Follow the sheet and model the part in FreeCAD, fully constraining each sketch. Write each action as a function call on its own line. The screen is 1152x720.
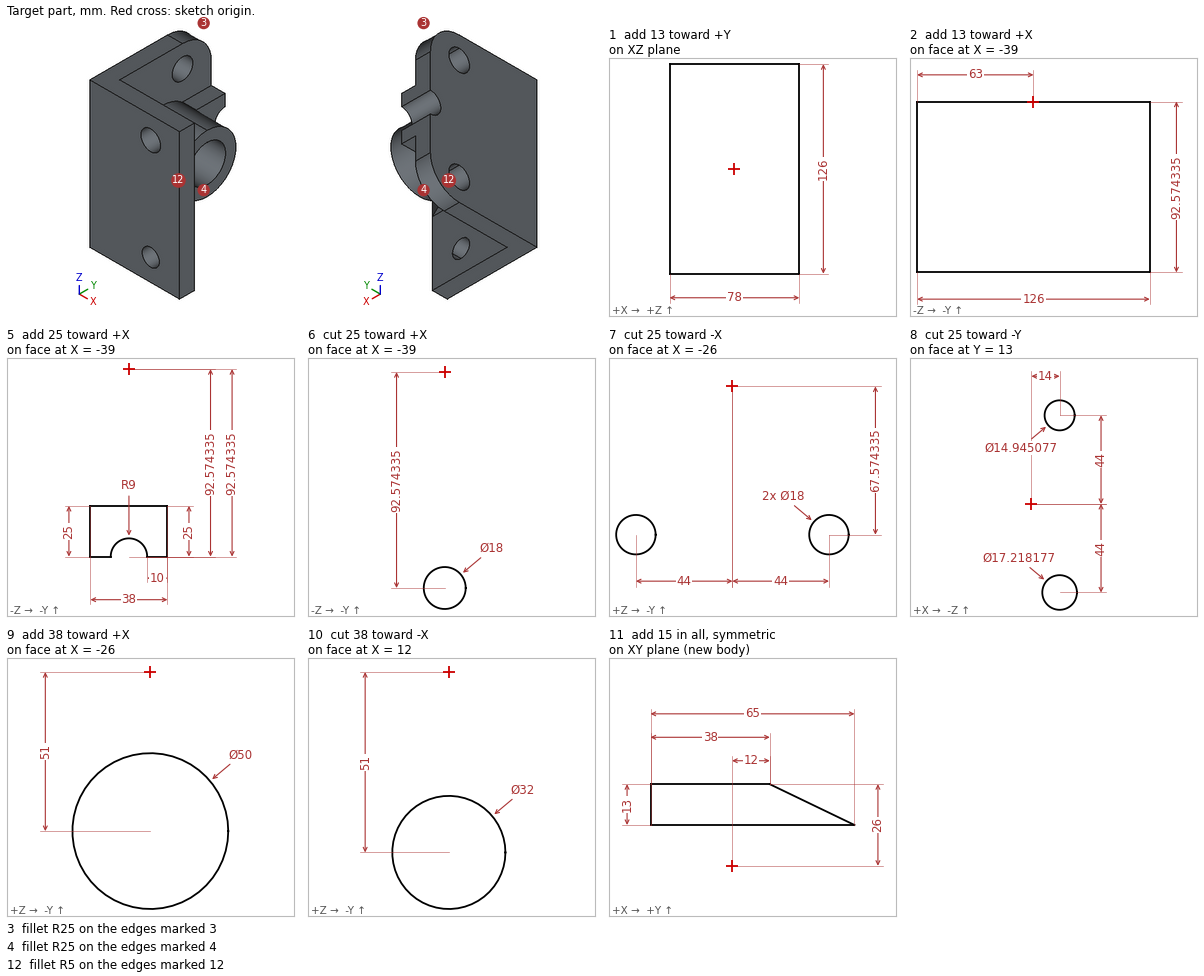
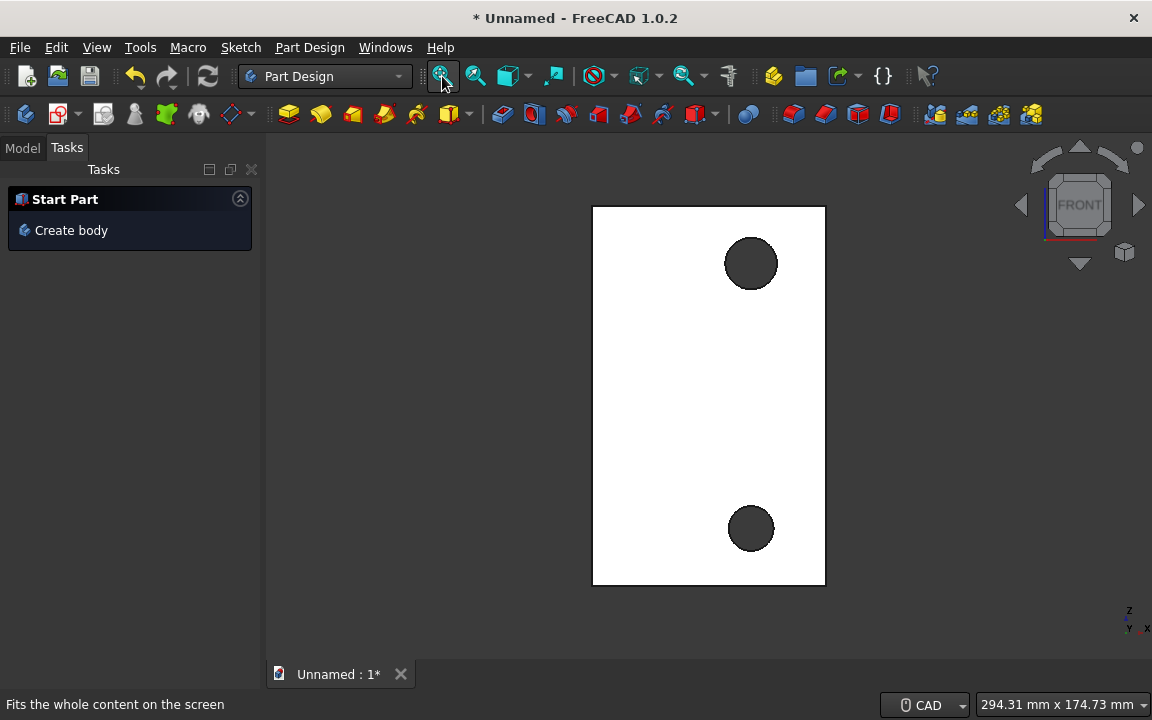
key(3)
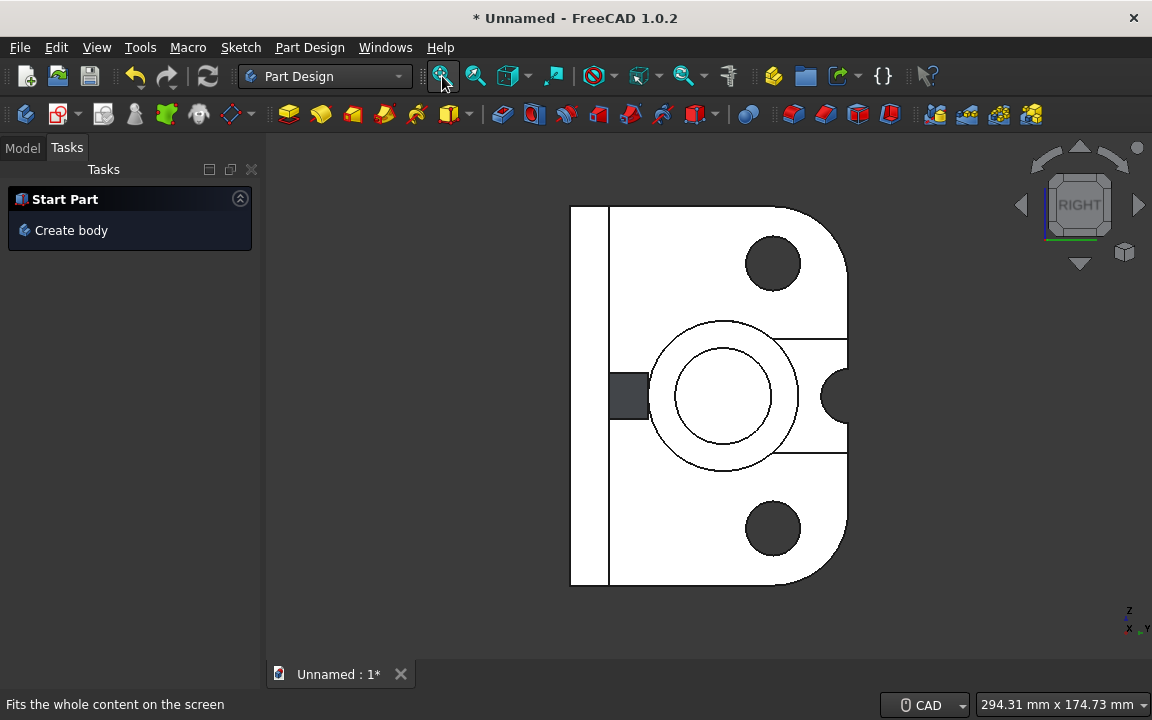
key(v)
key(f)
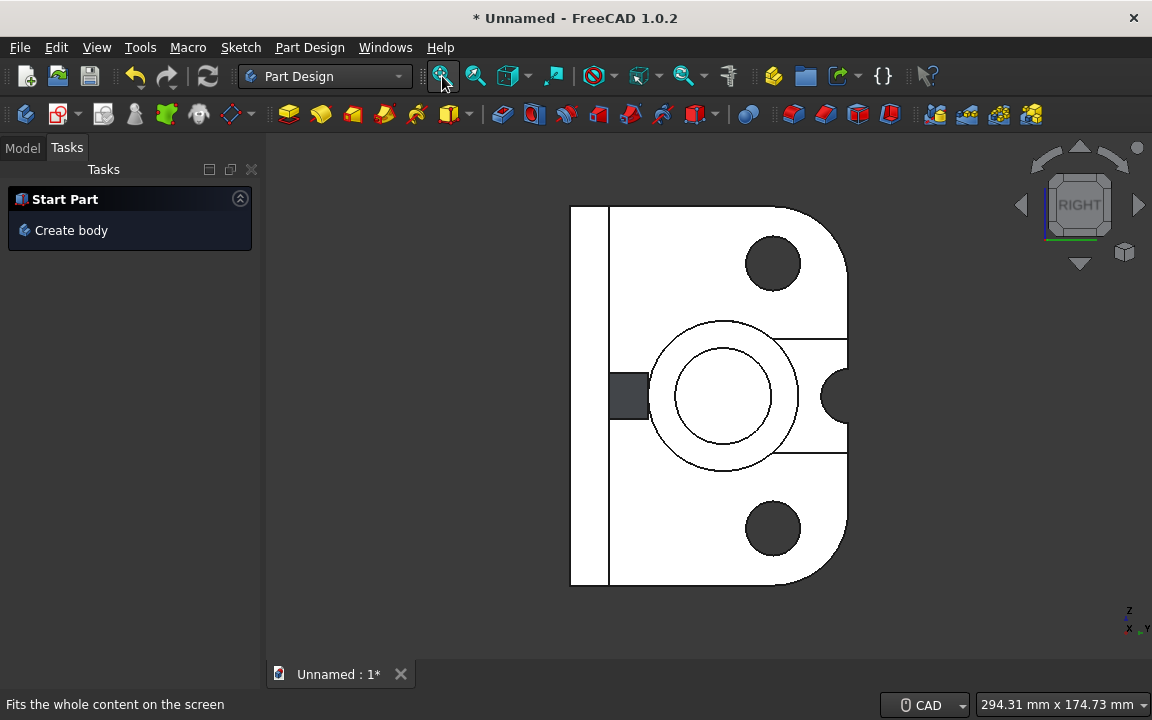
key(5)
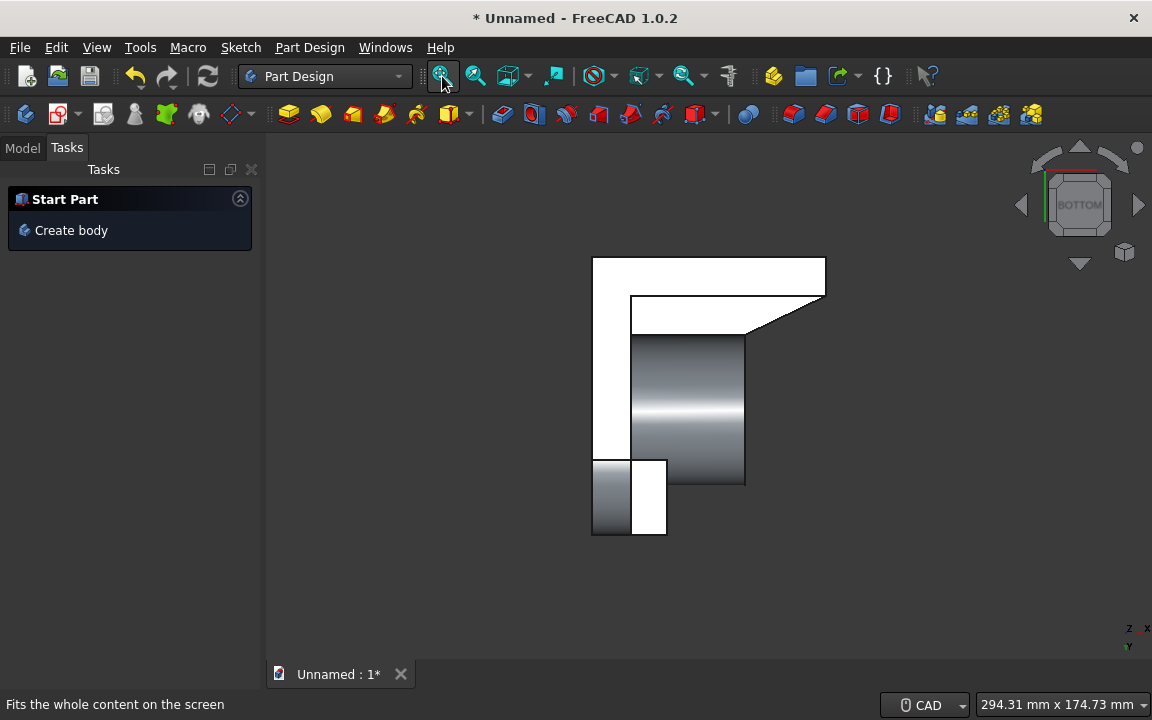
key(v)
key(f)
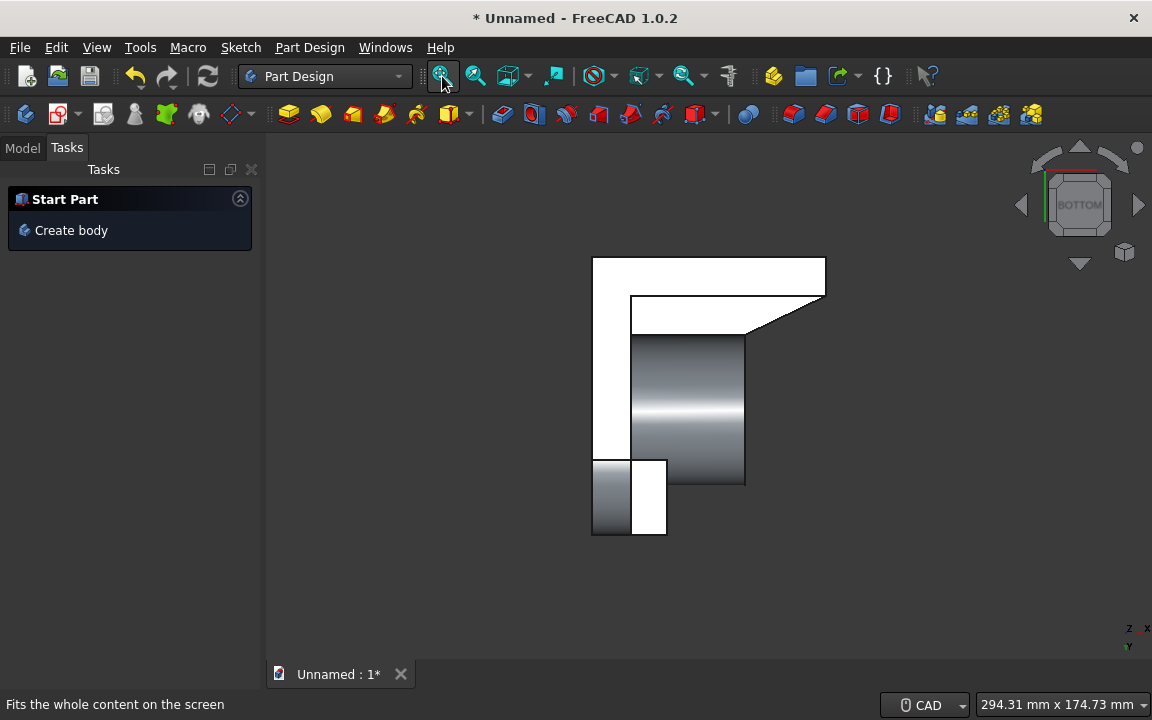
key(4)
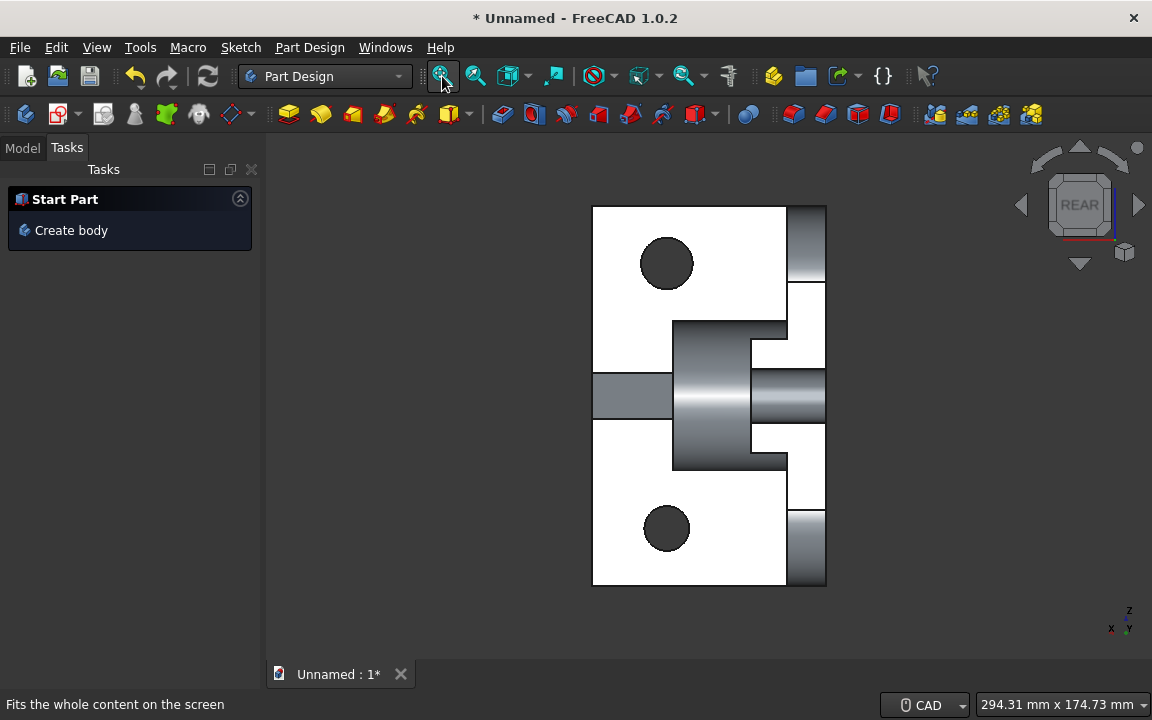
key(v)
key(f)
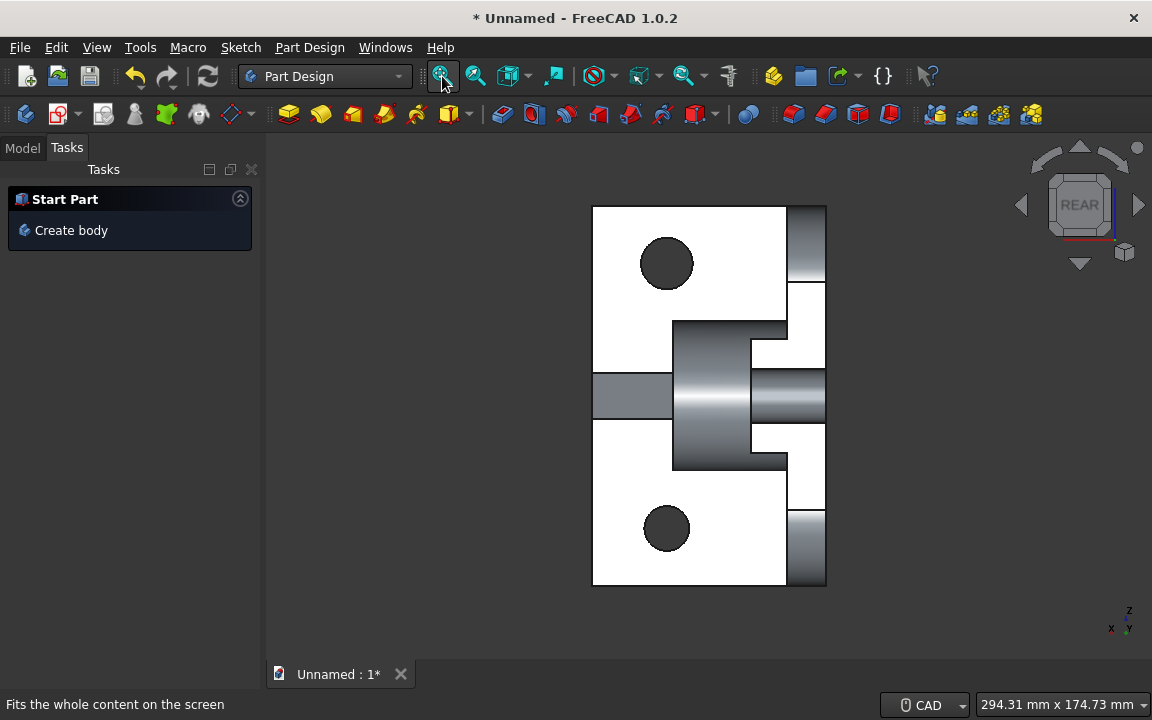
key(6)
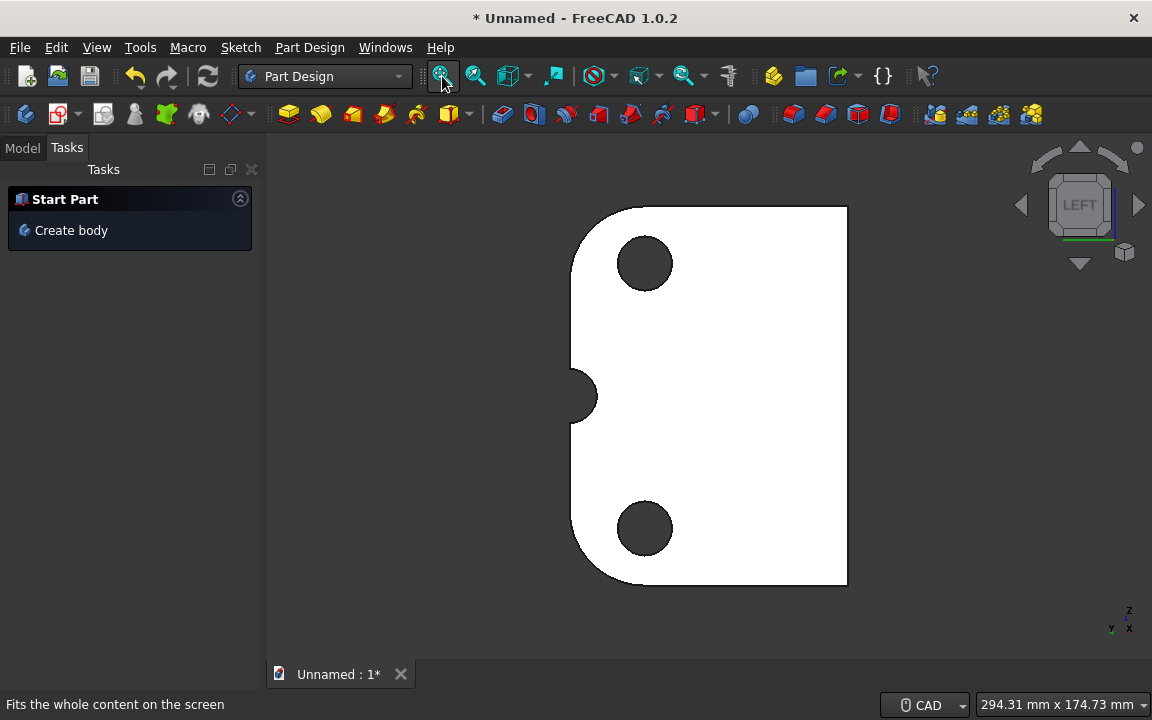
key(v)
key(f)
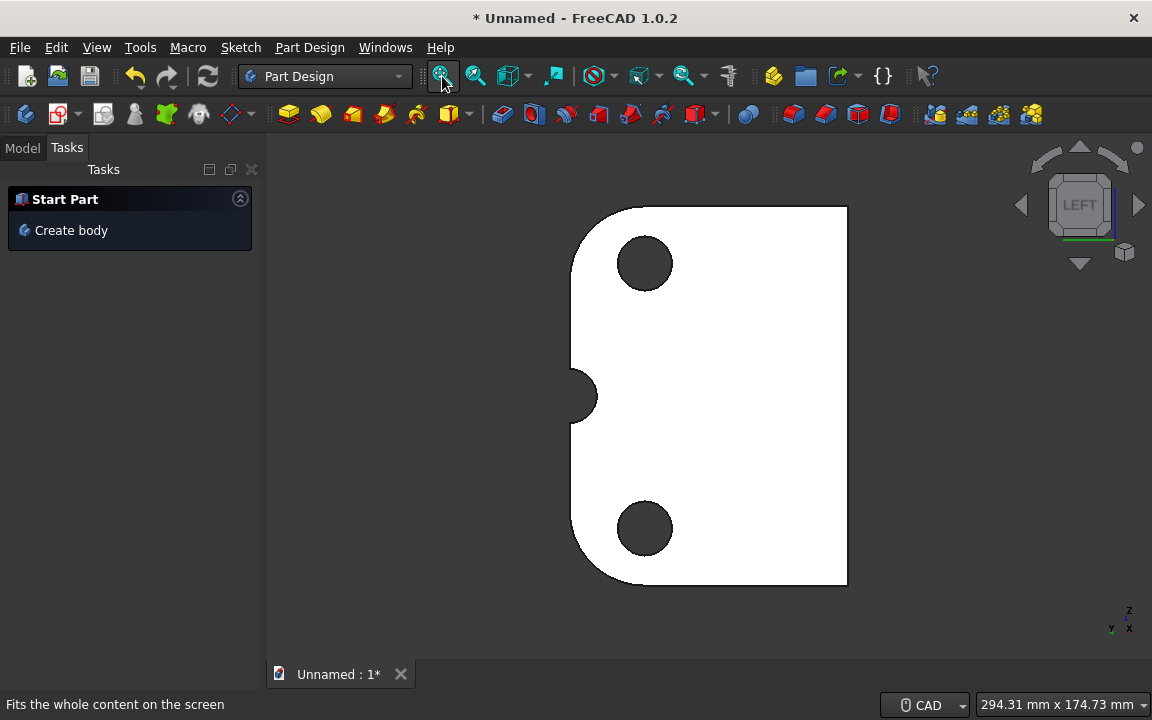
key(v)
key(3)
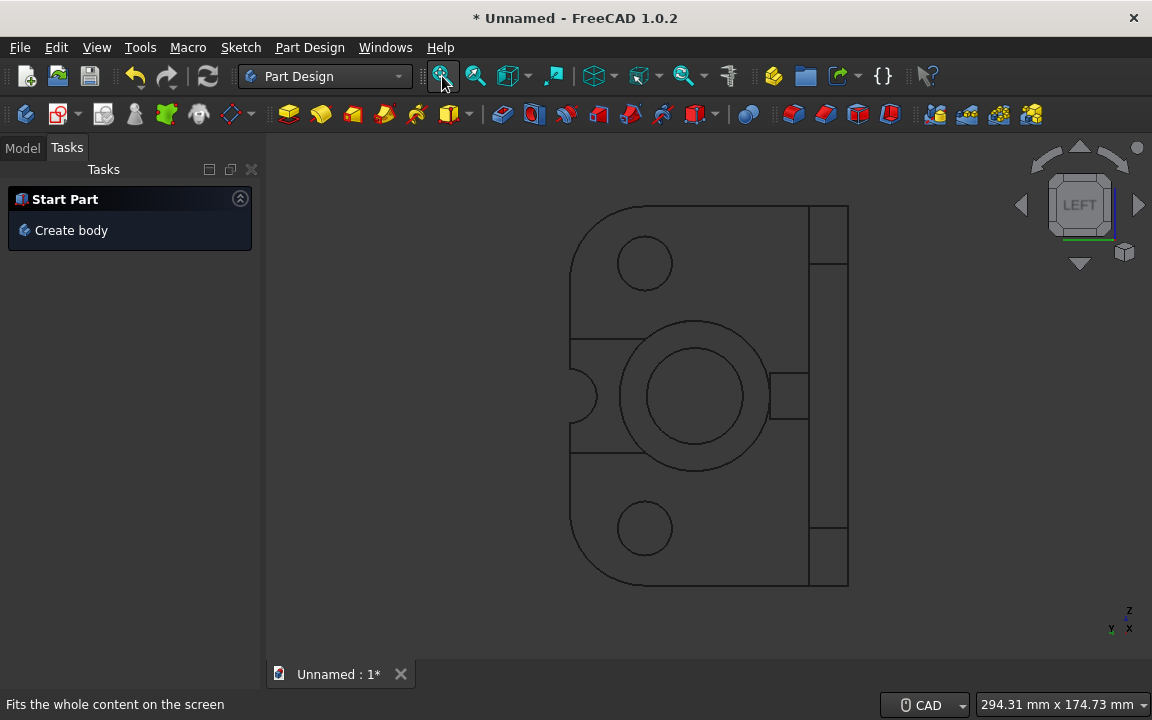
key(0)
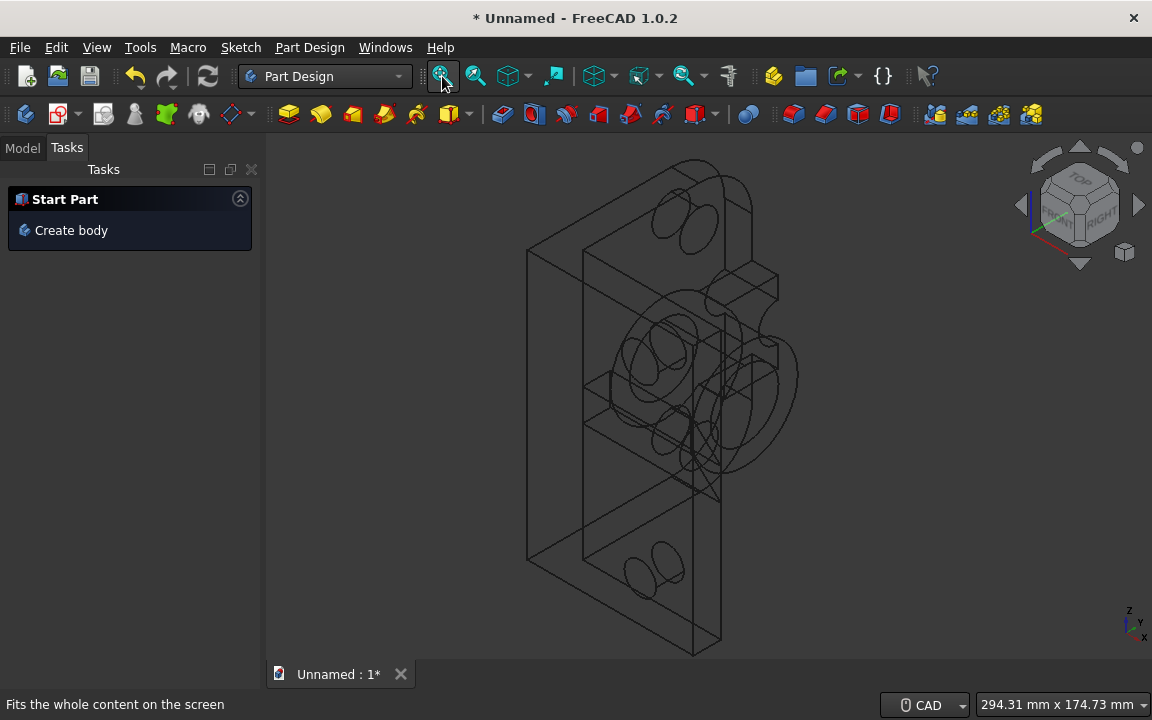
click(444, 76)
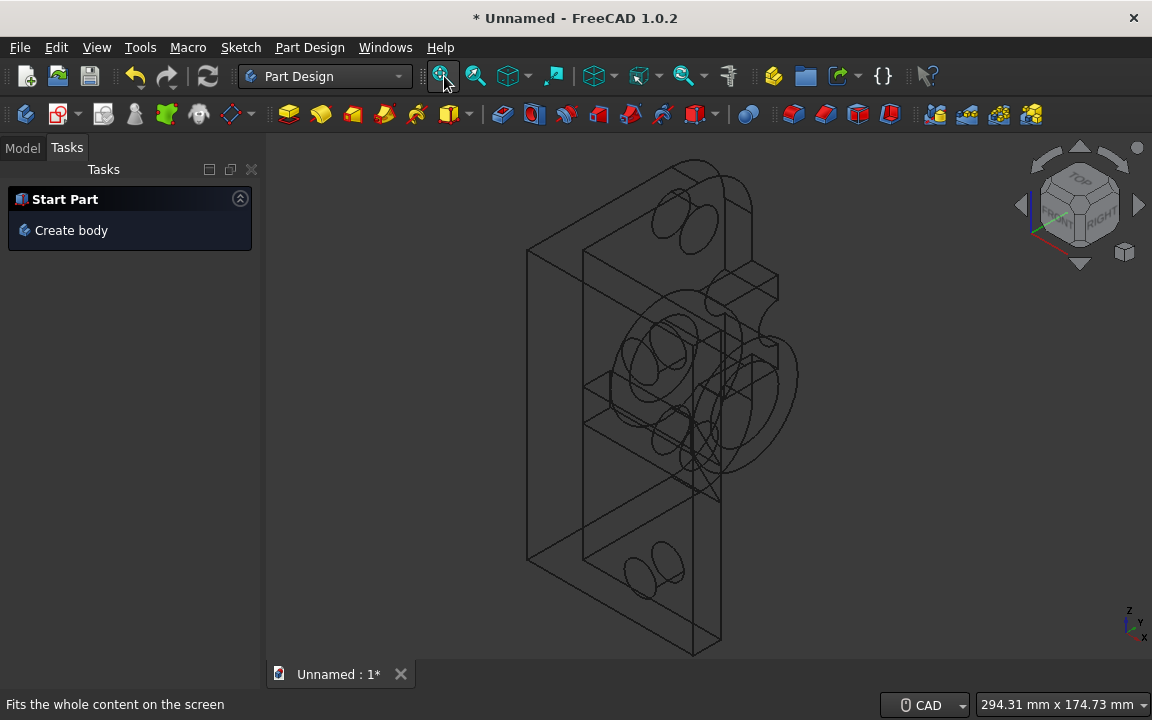
key(2)